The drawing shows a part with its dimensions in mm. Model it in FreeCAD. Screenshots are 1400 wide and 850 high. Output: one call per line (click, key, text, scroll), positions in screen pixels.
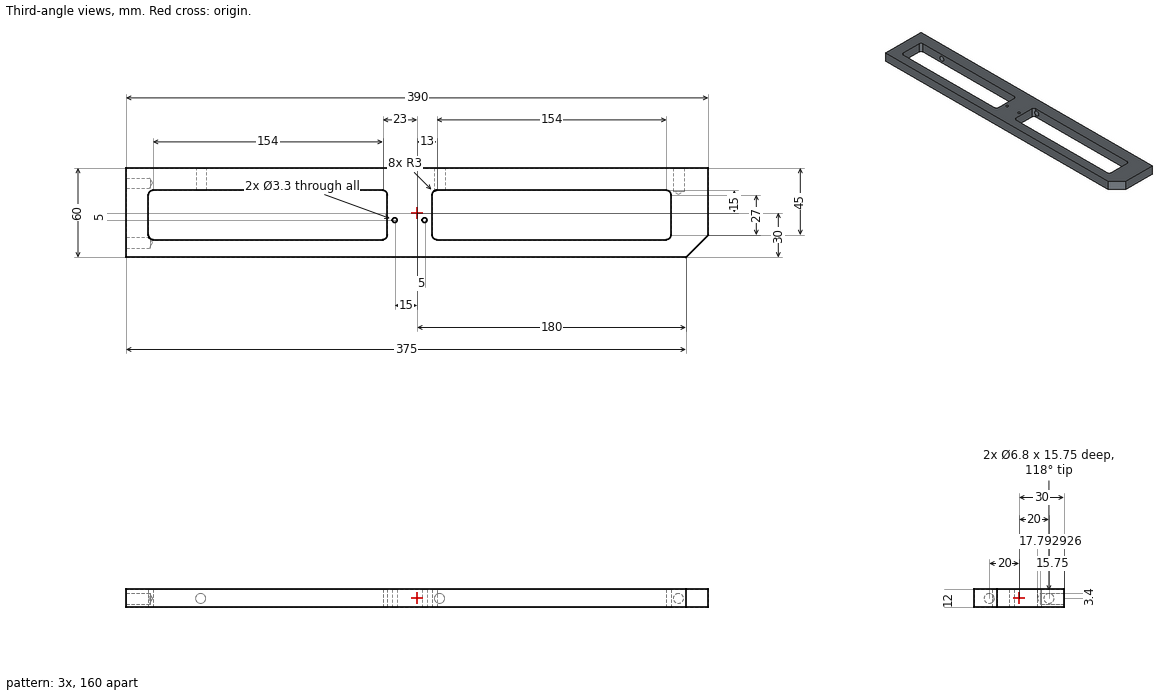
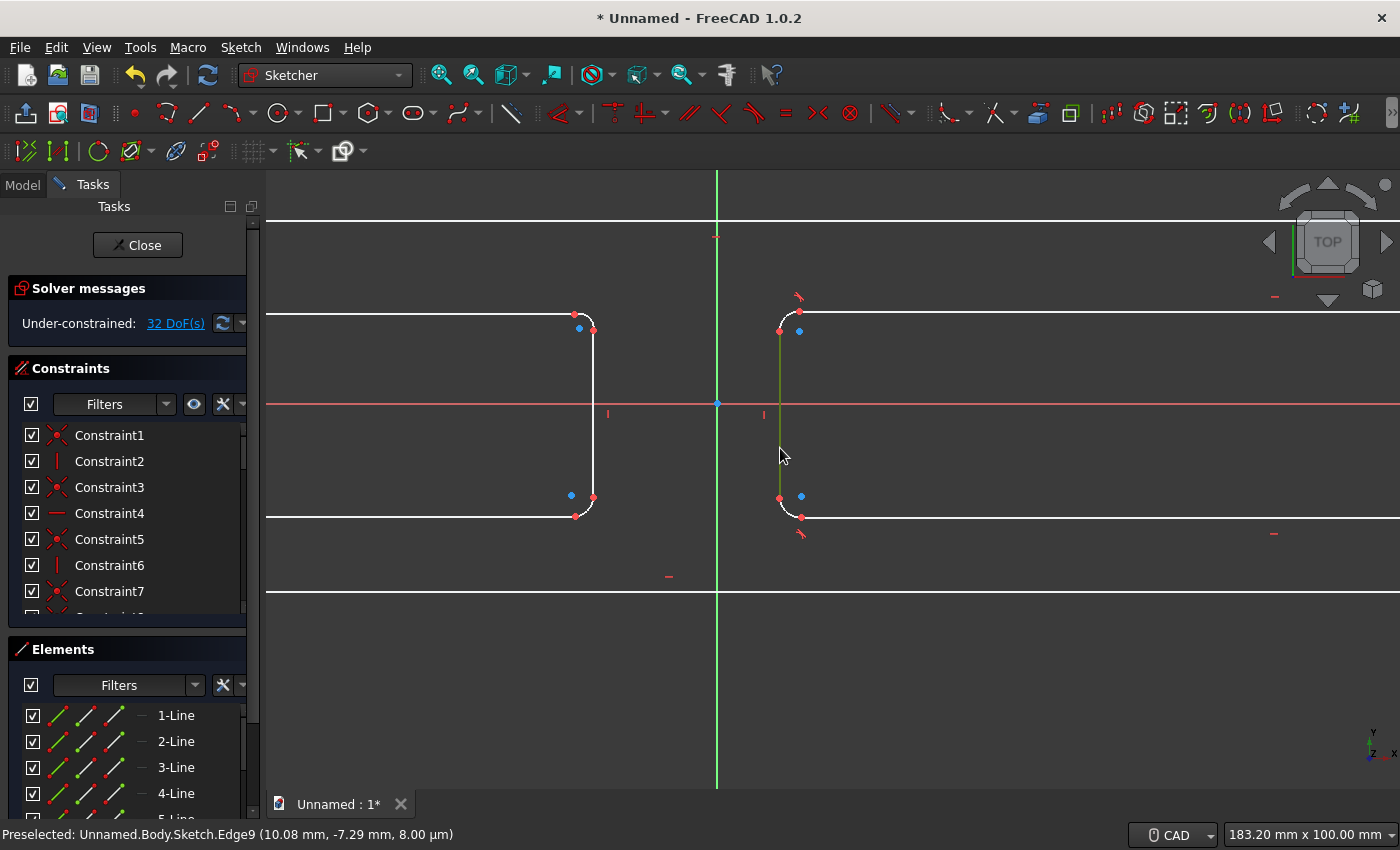
scroll(783, 507, up, 2)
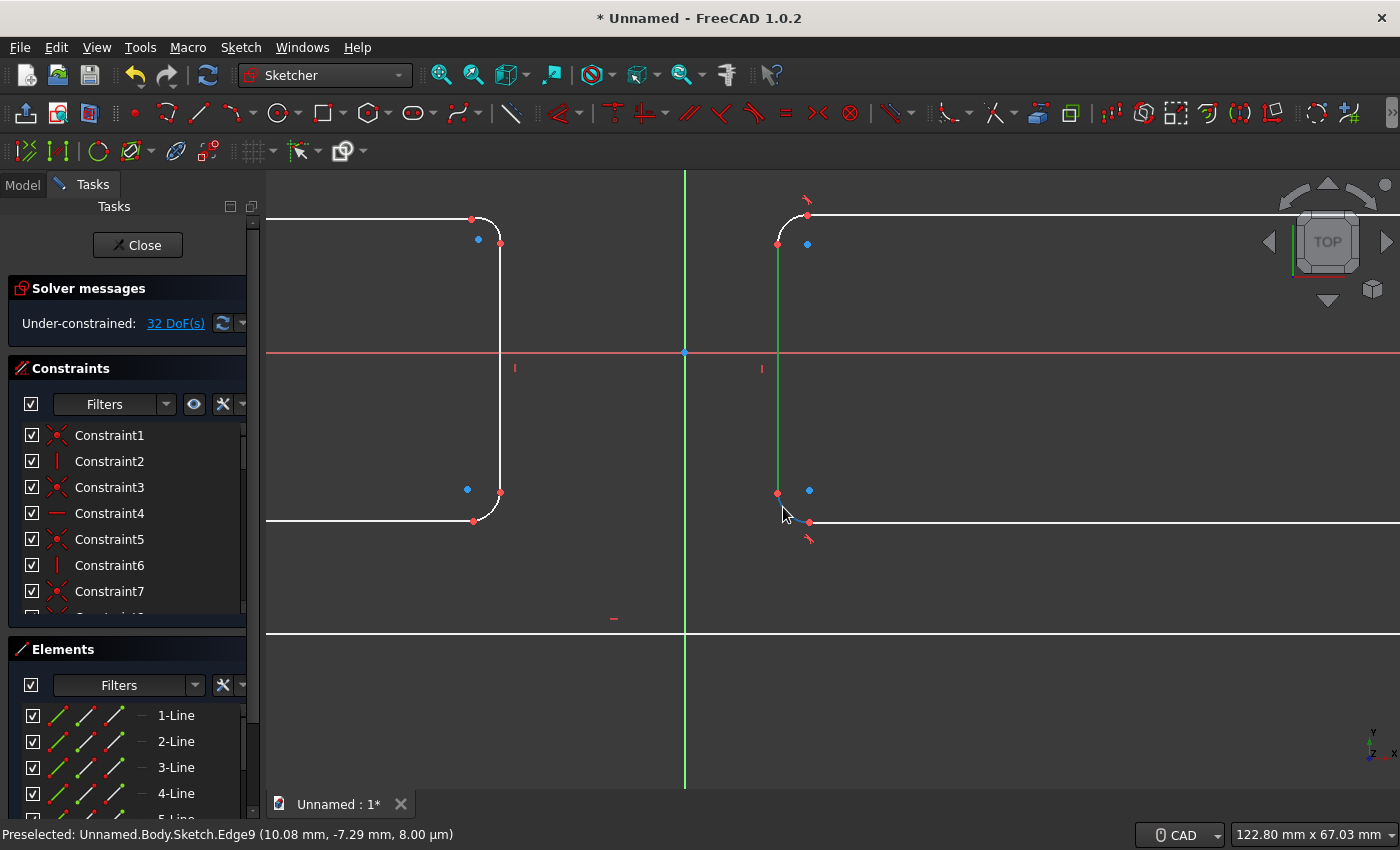
click(782, 507)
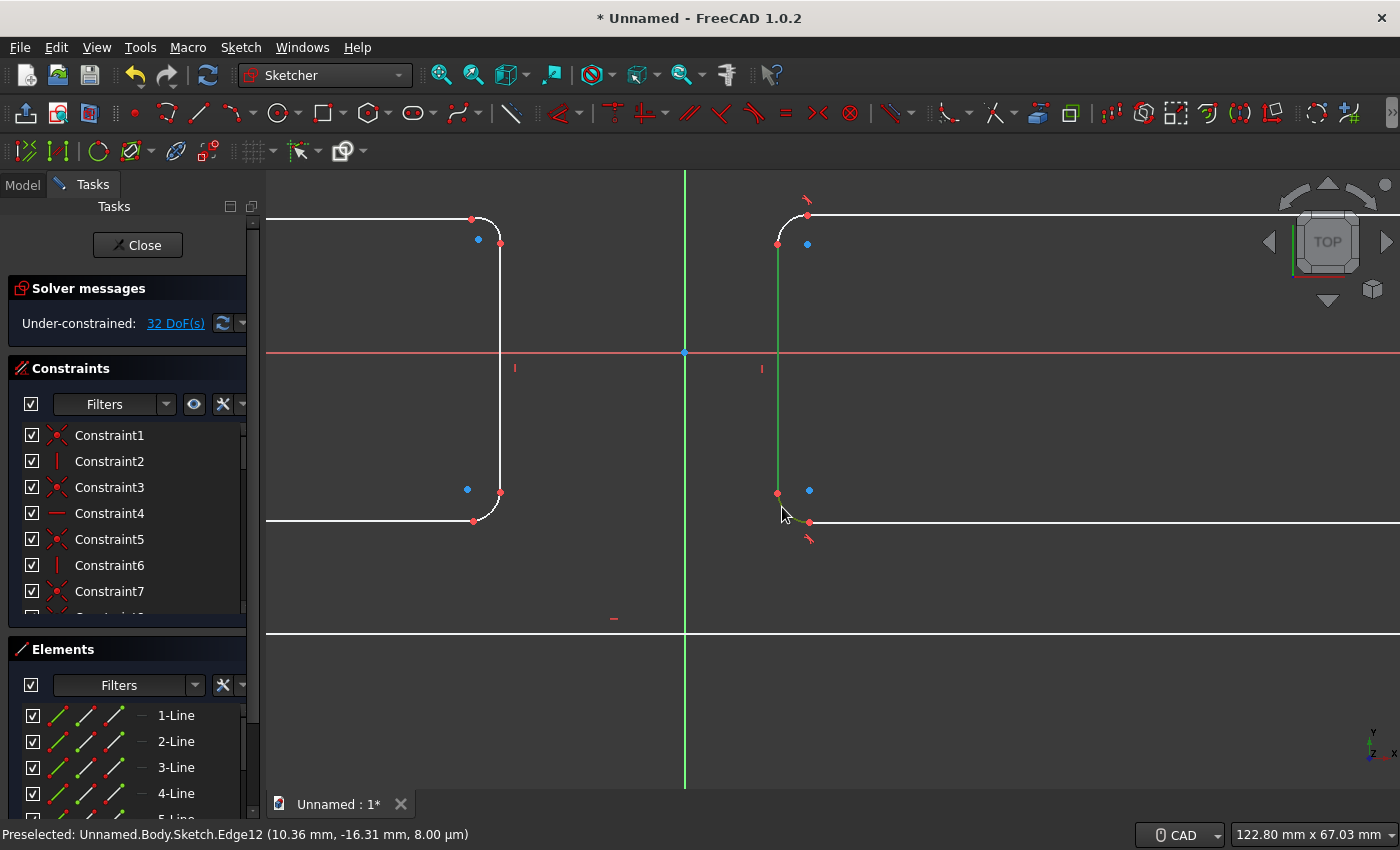
click(754, 114)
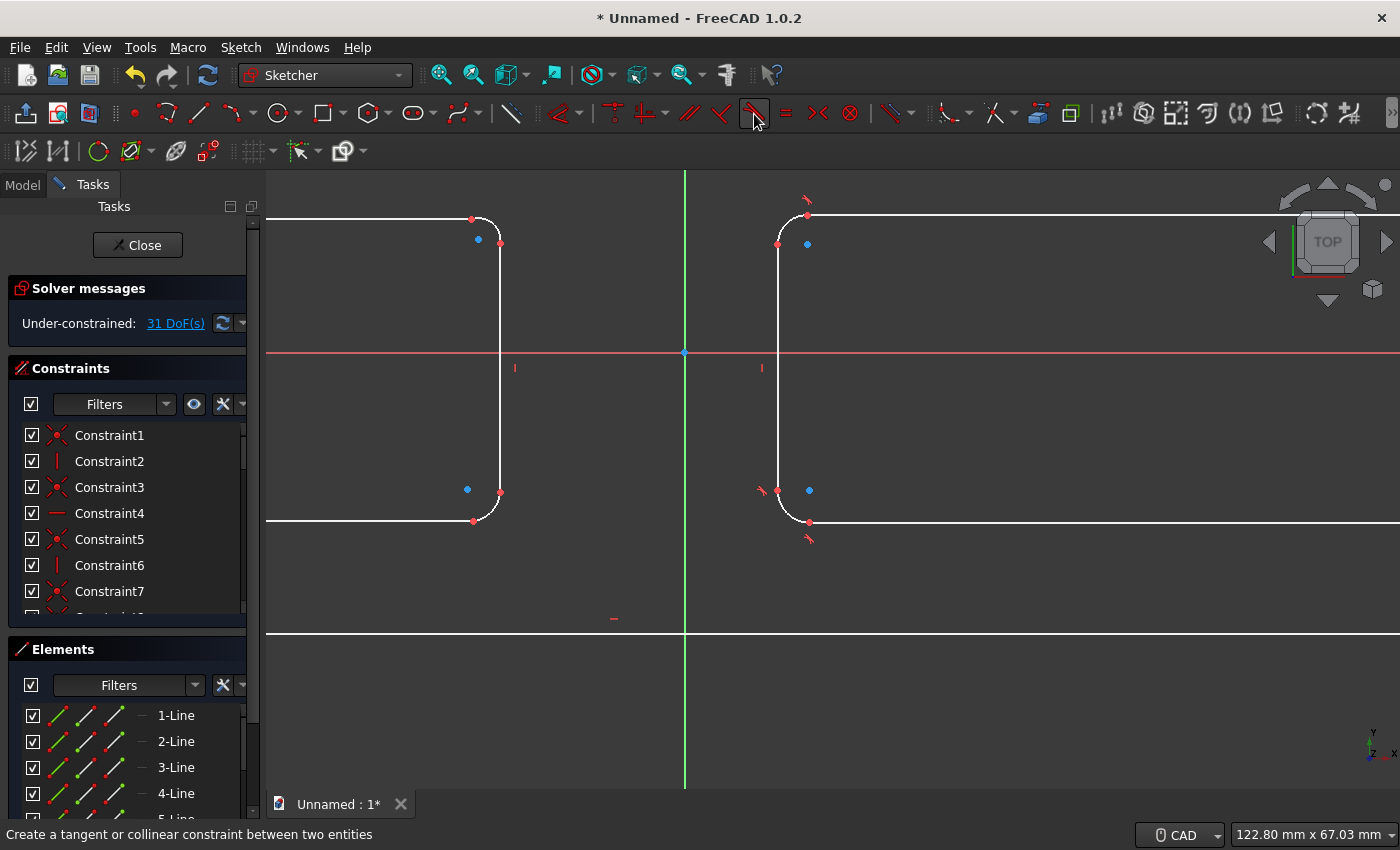
scroll(785, 512, down, 8)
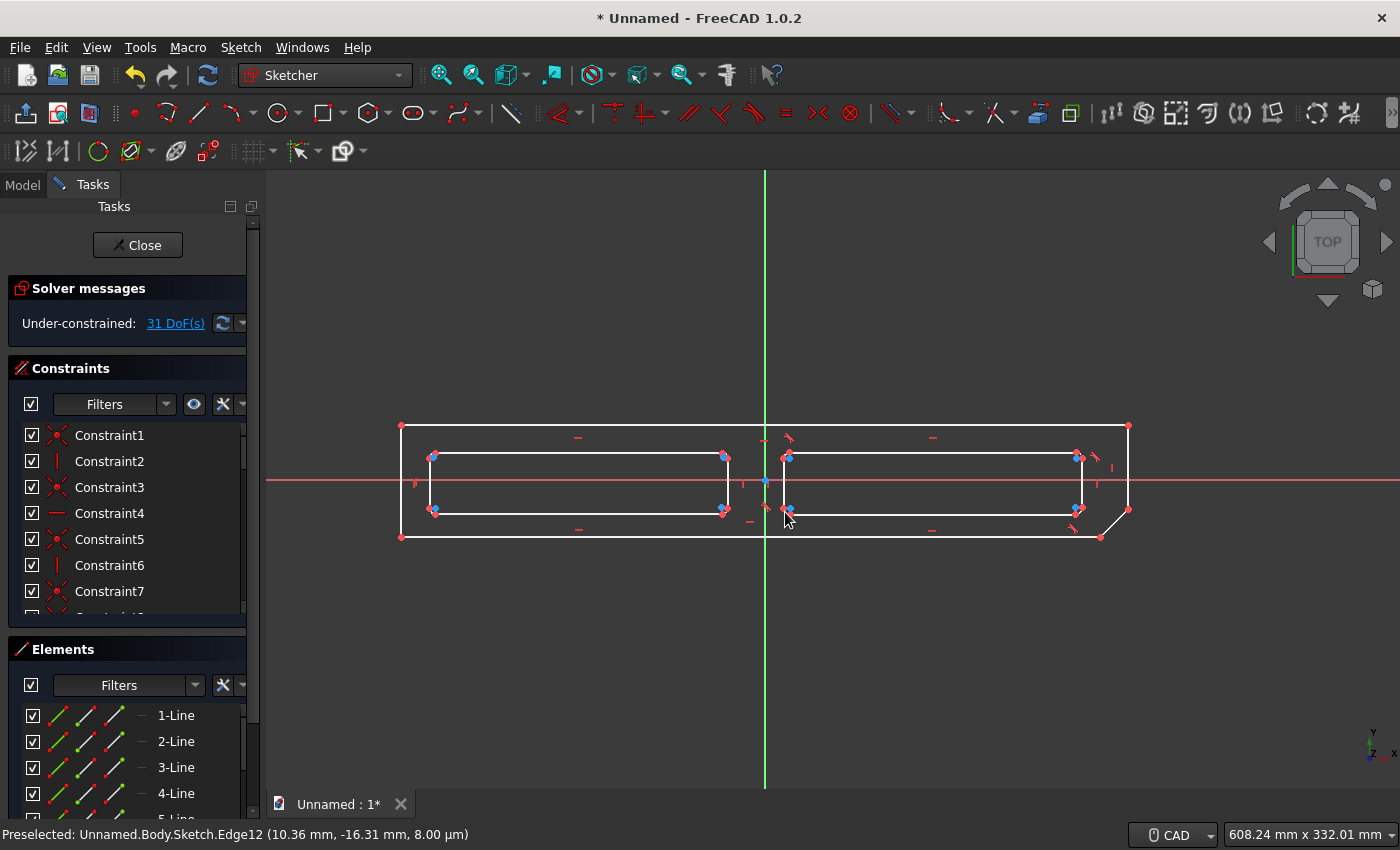
click(784, 493)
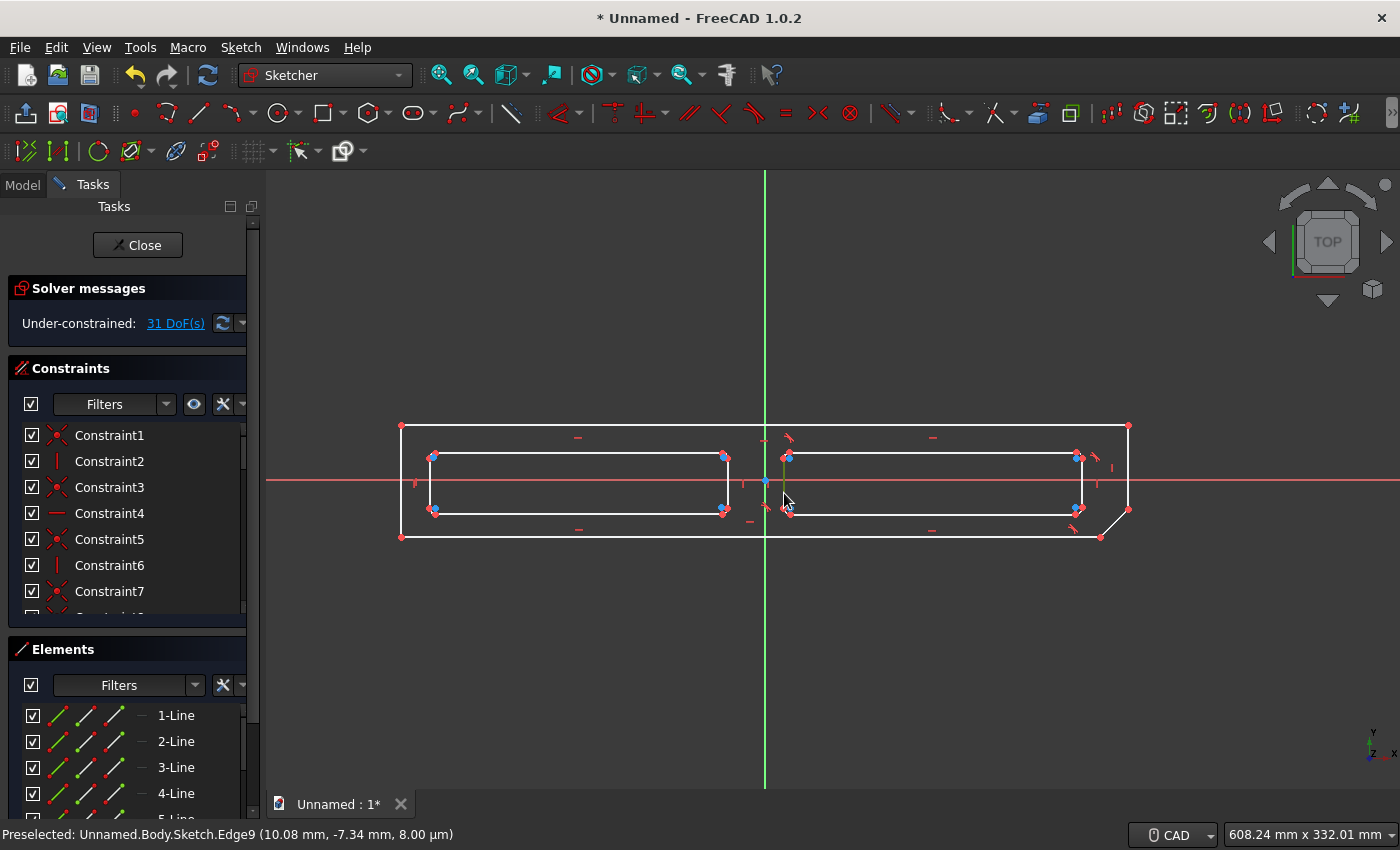
scroll(786, 454, up, 6)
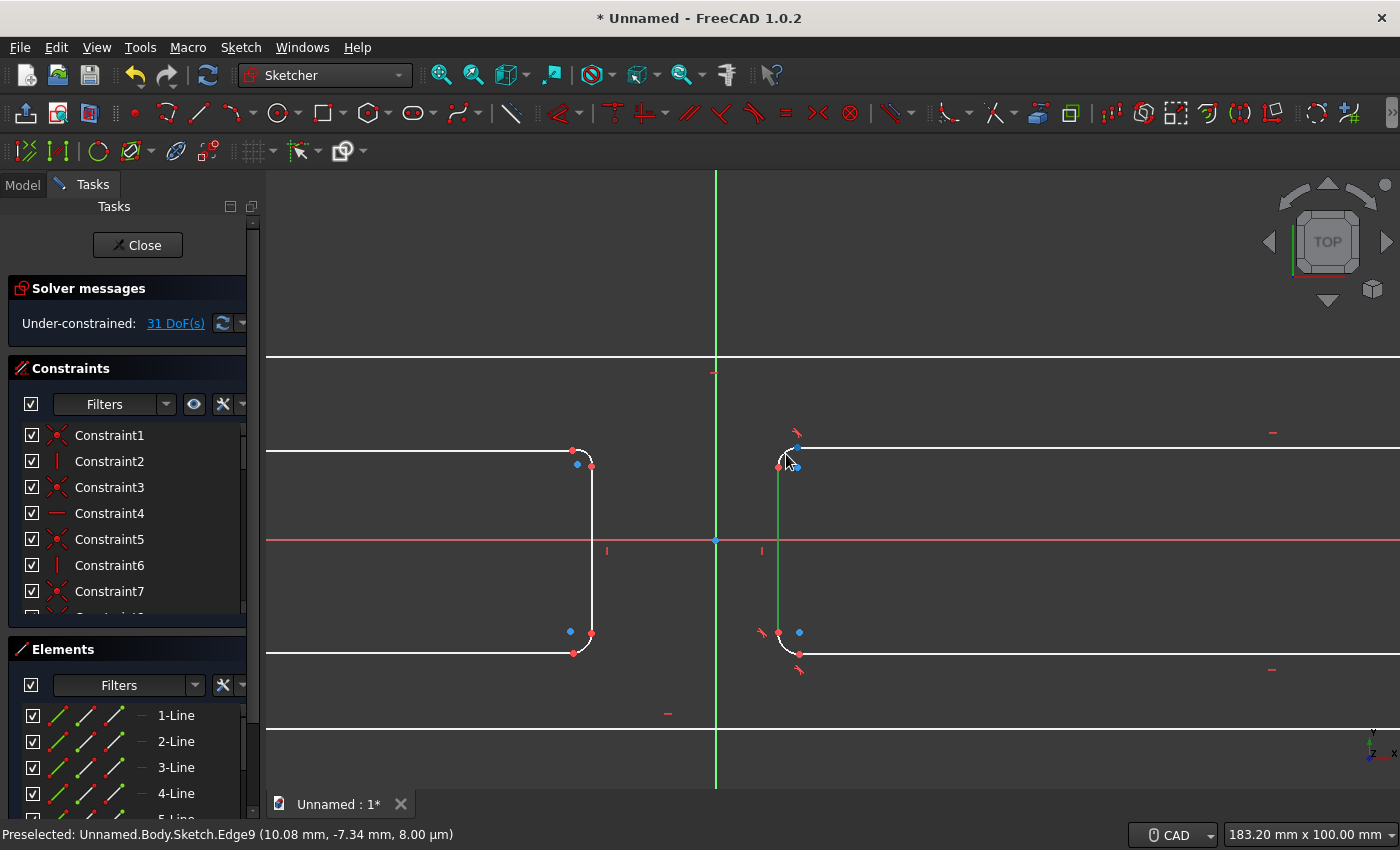
click(784, 454)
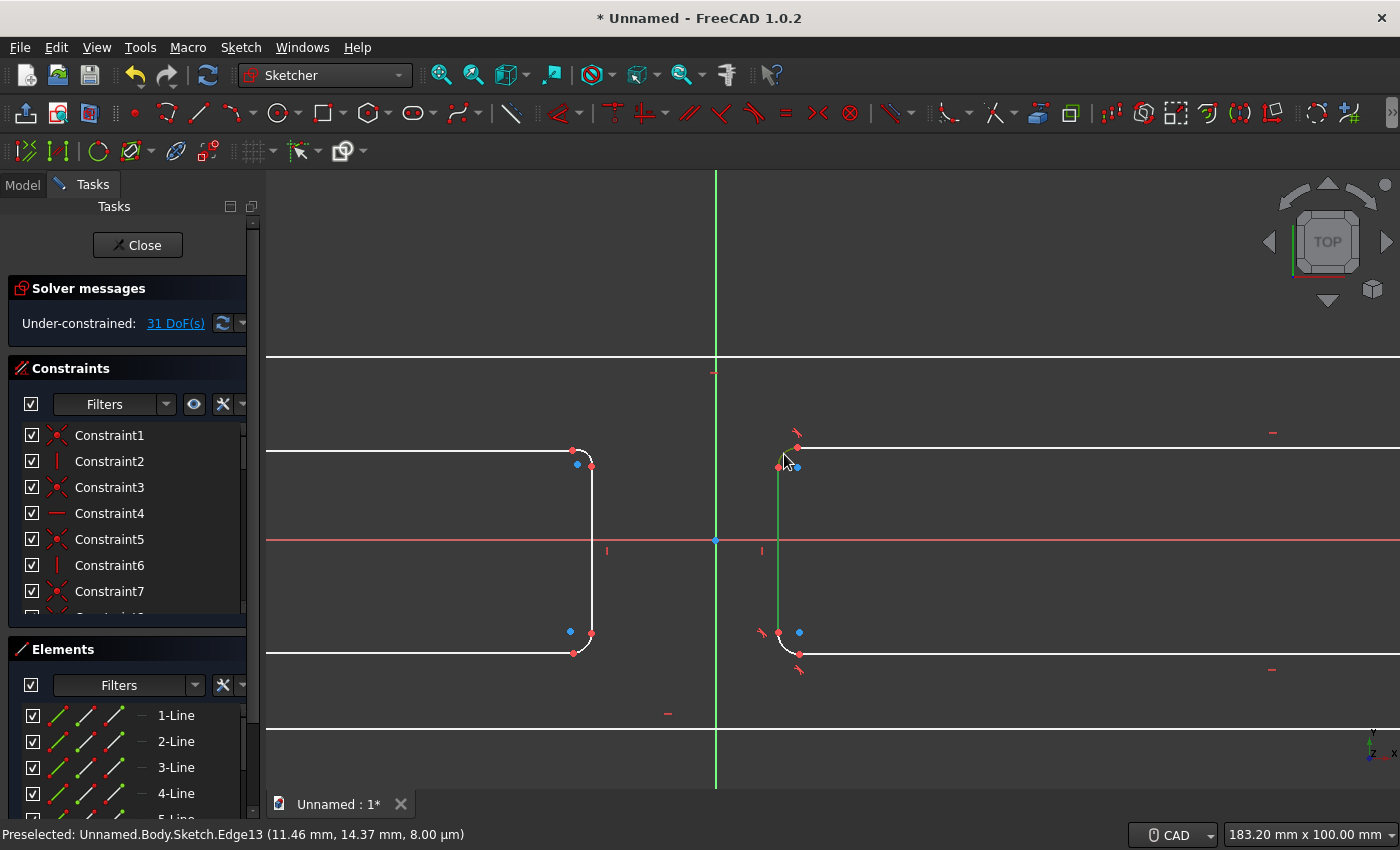
click(754, 114)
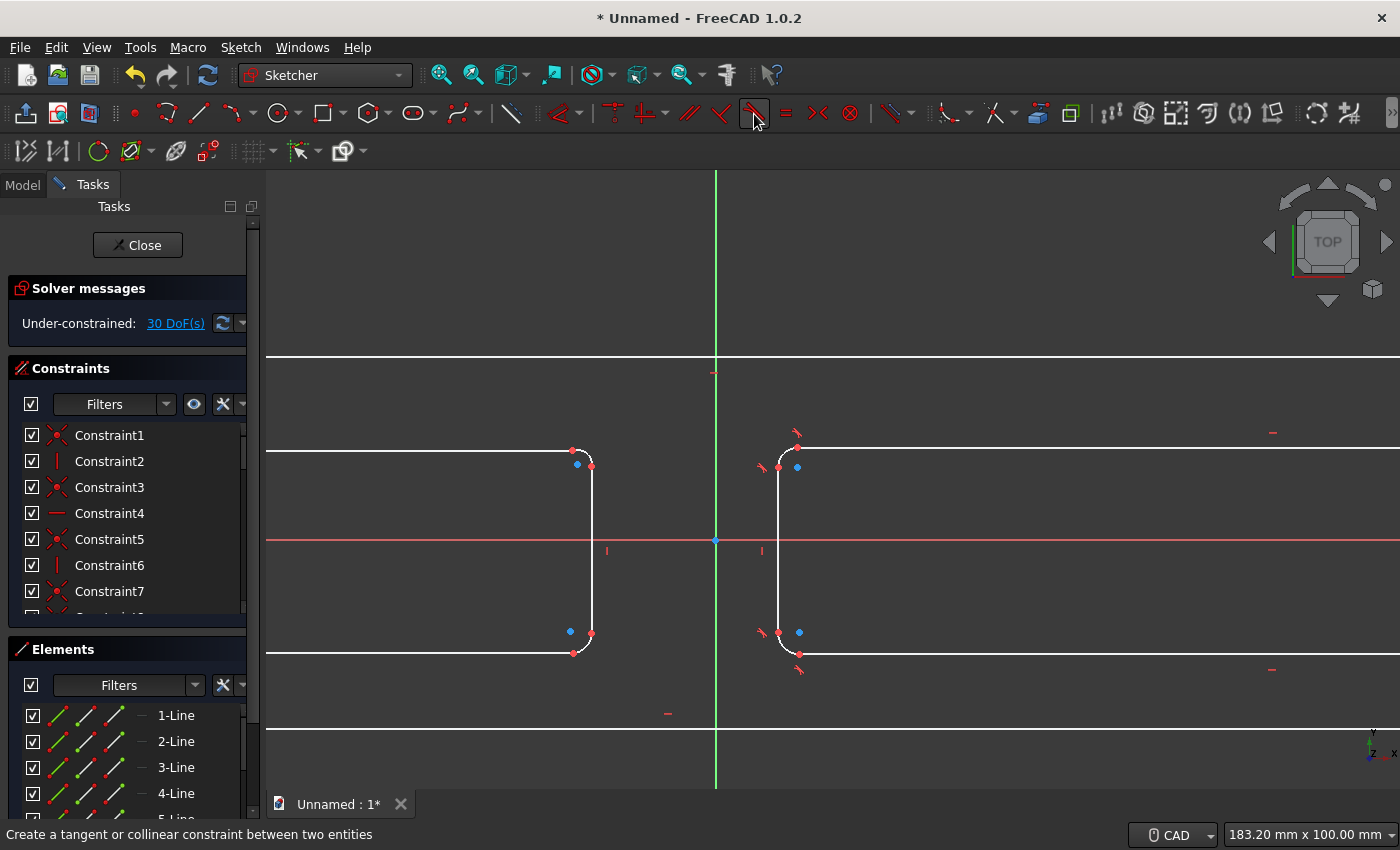
click(382, 451)